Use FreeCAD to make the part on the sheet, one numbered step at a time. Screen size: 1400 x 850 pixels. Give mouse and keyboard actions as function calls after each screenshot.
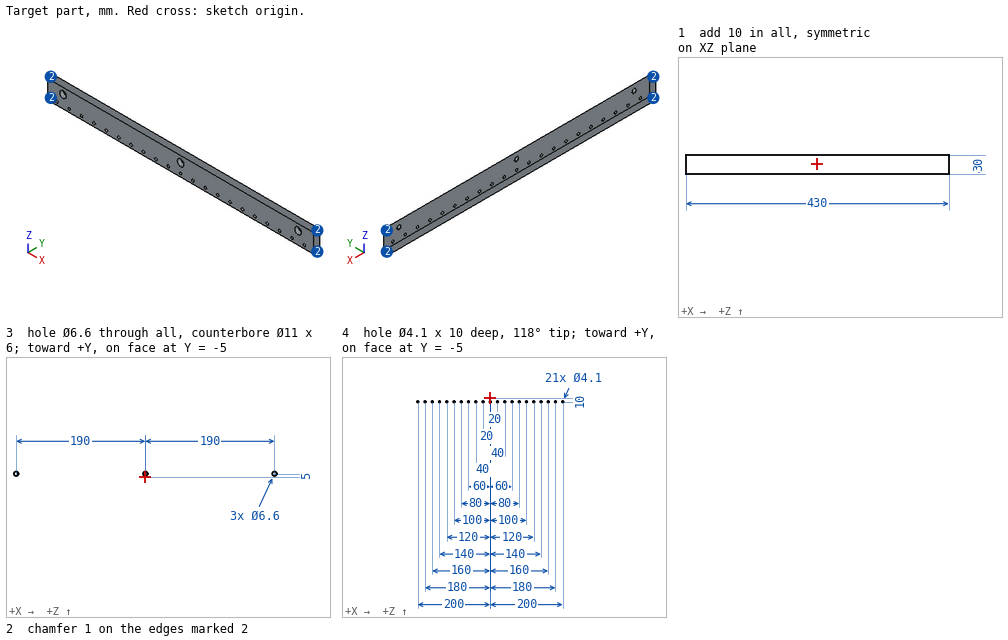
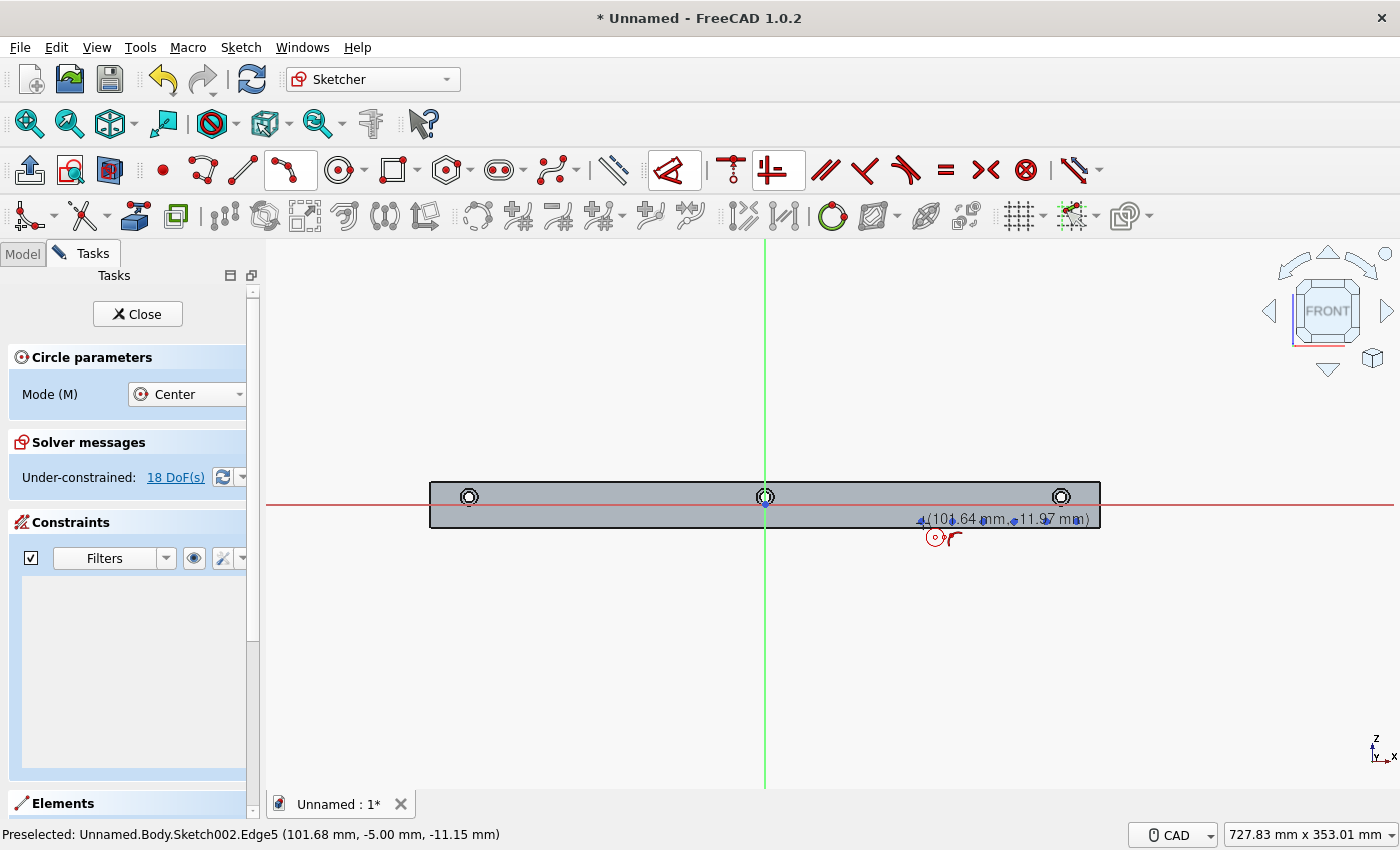
click(890, 521)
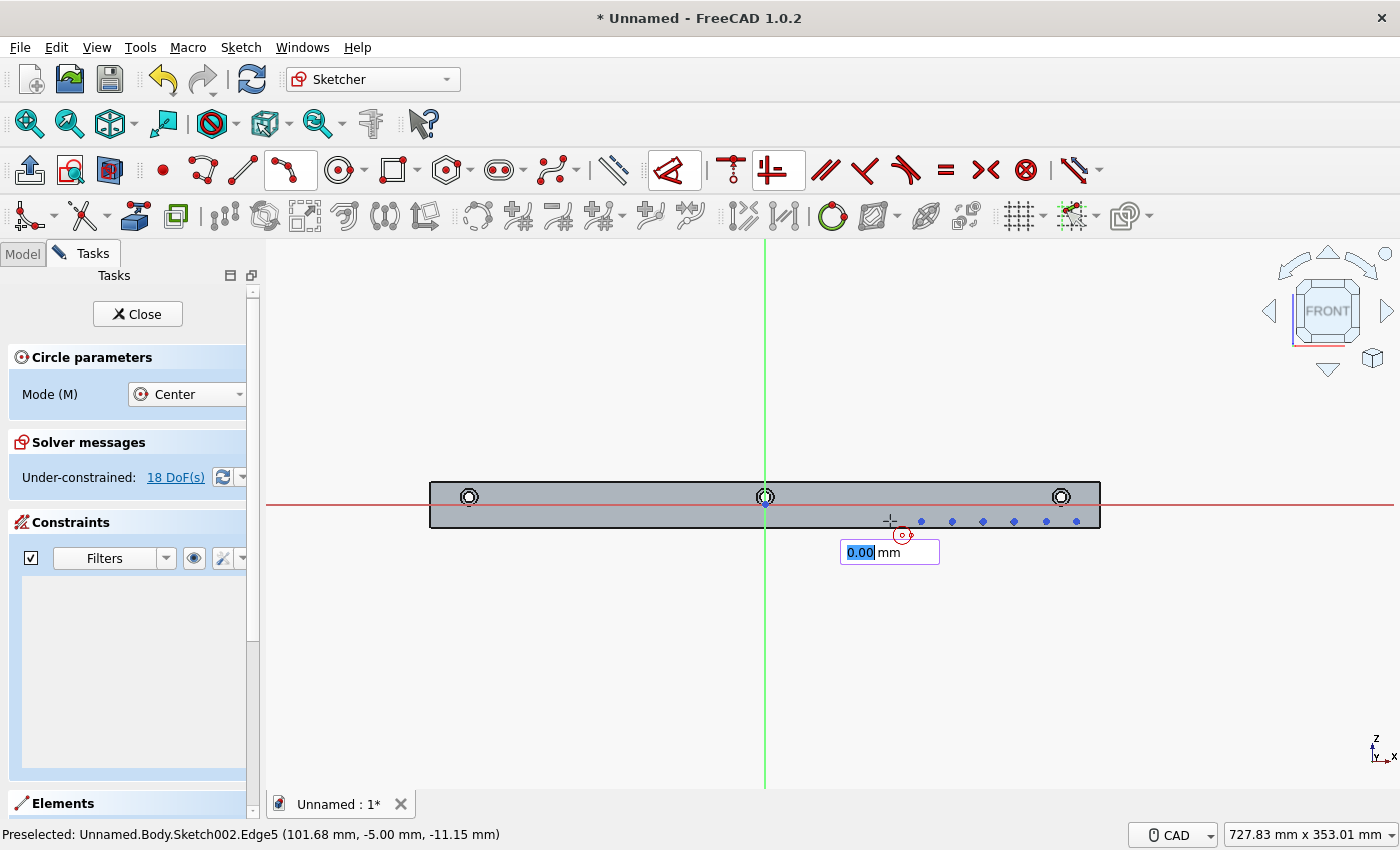
scroll(892, 523, up, 9)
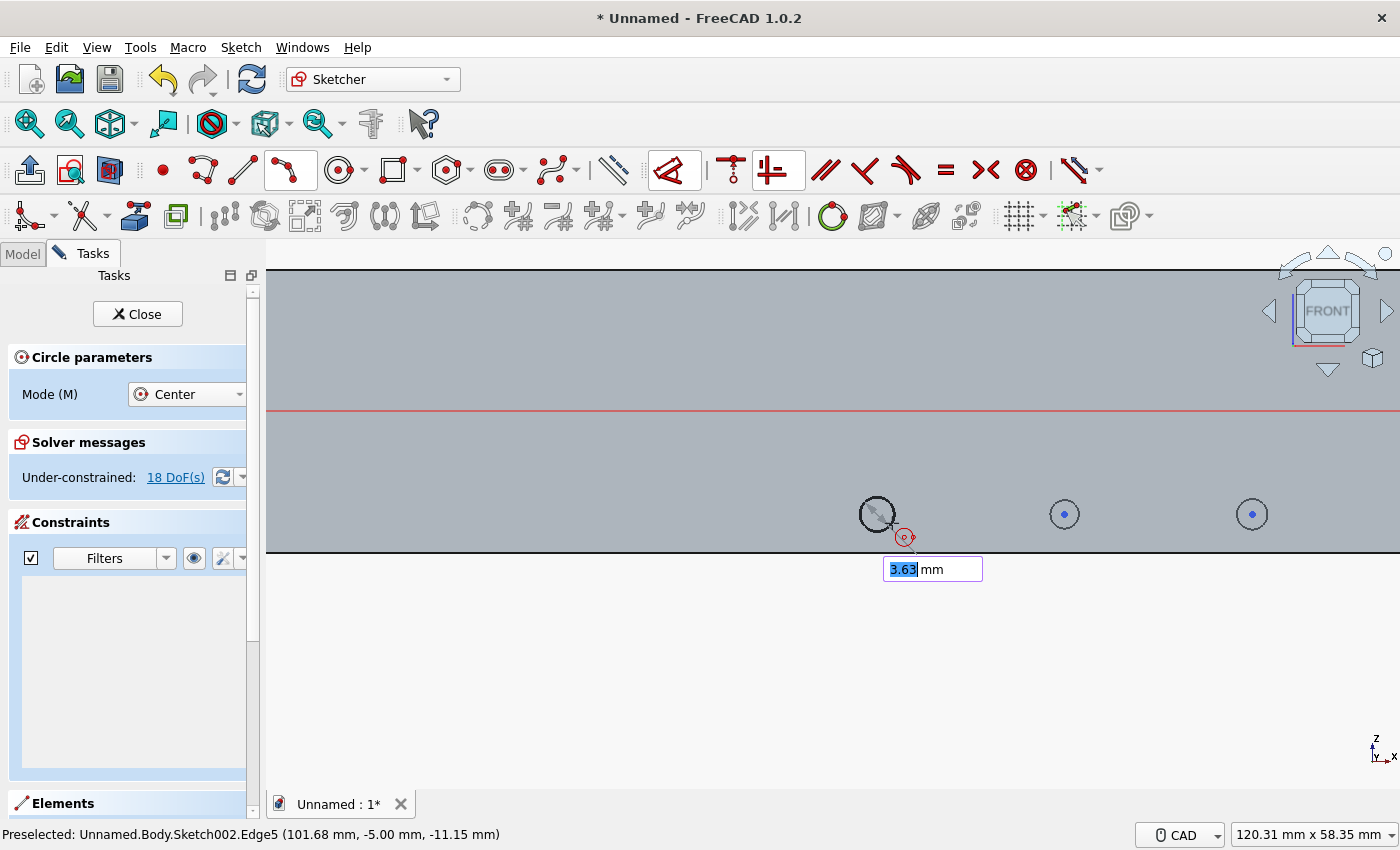
click(889, 519)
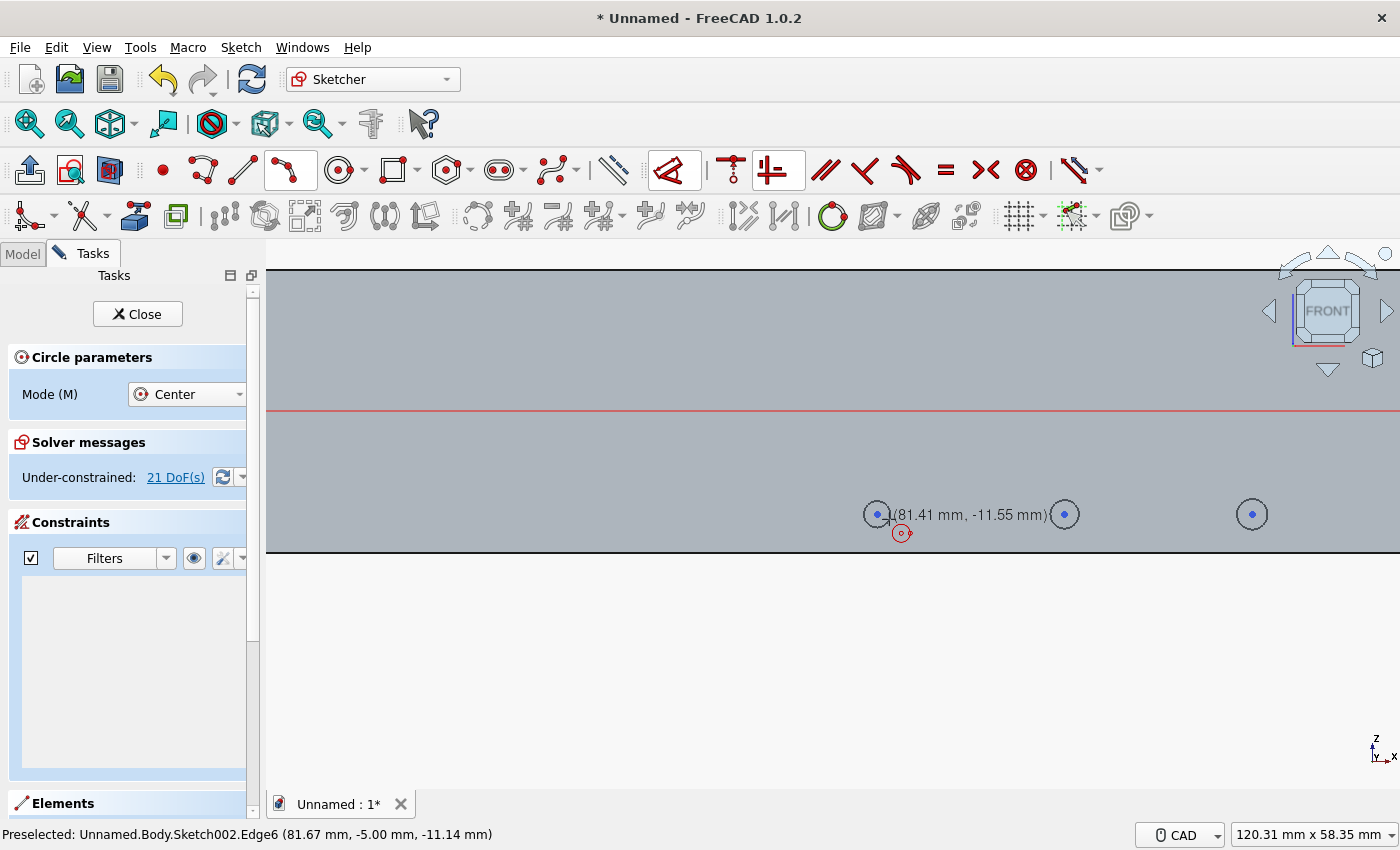
scroll(892, 523, down, 9)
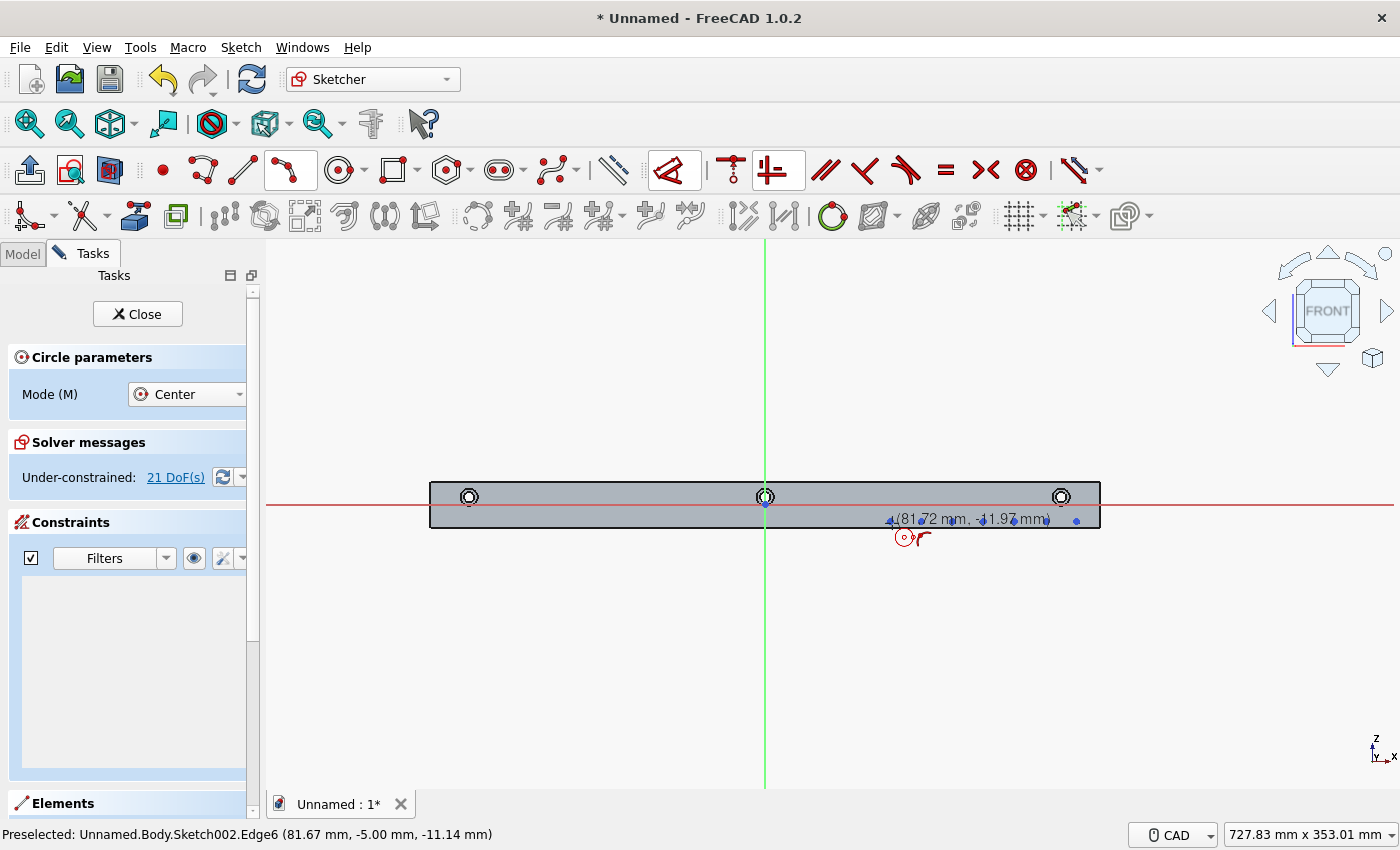
click(859, 521)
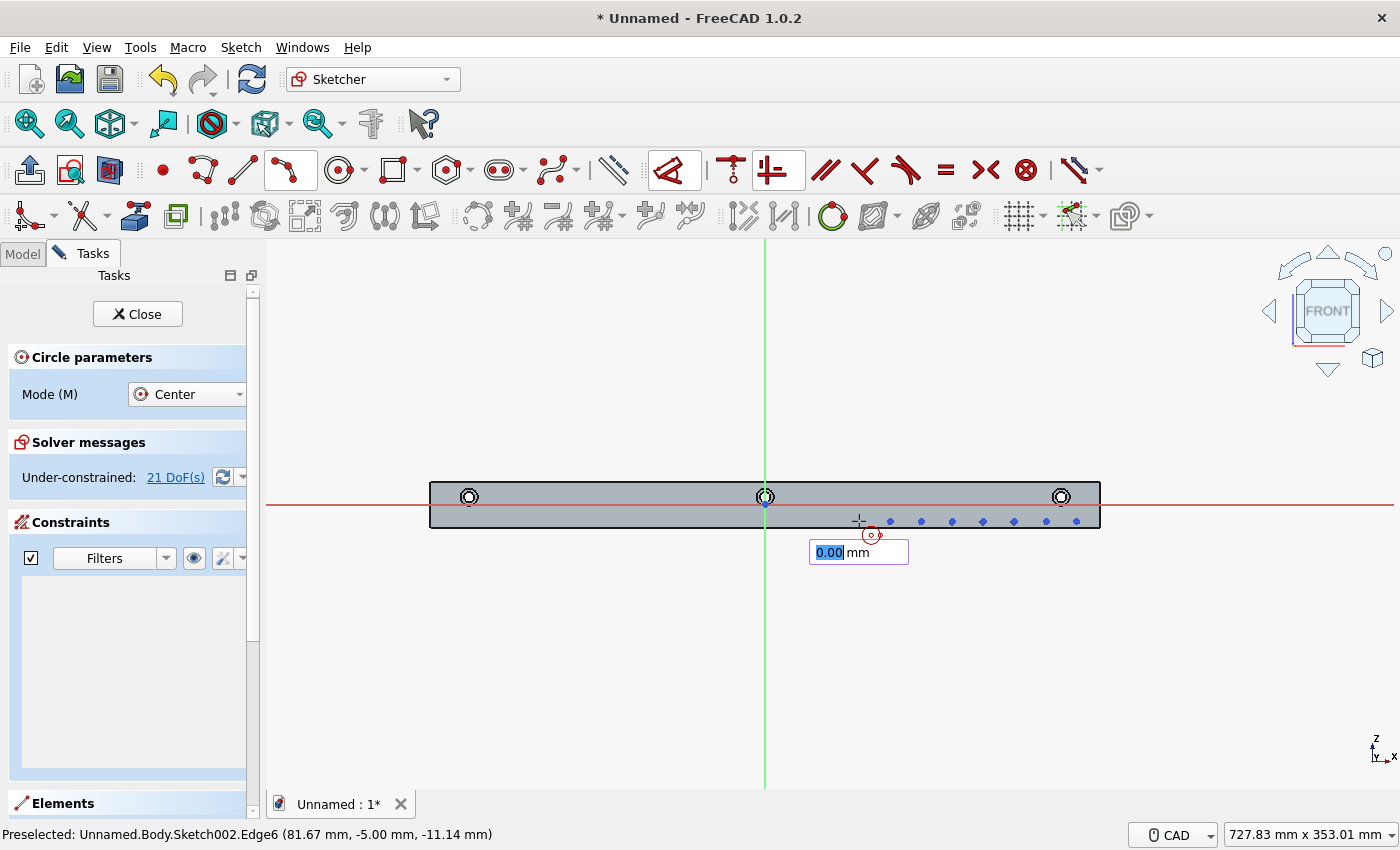
scroll(861, 523, up, 9)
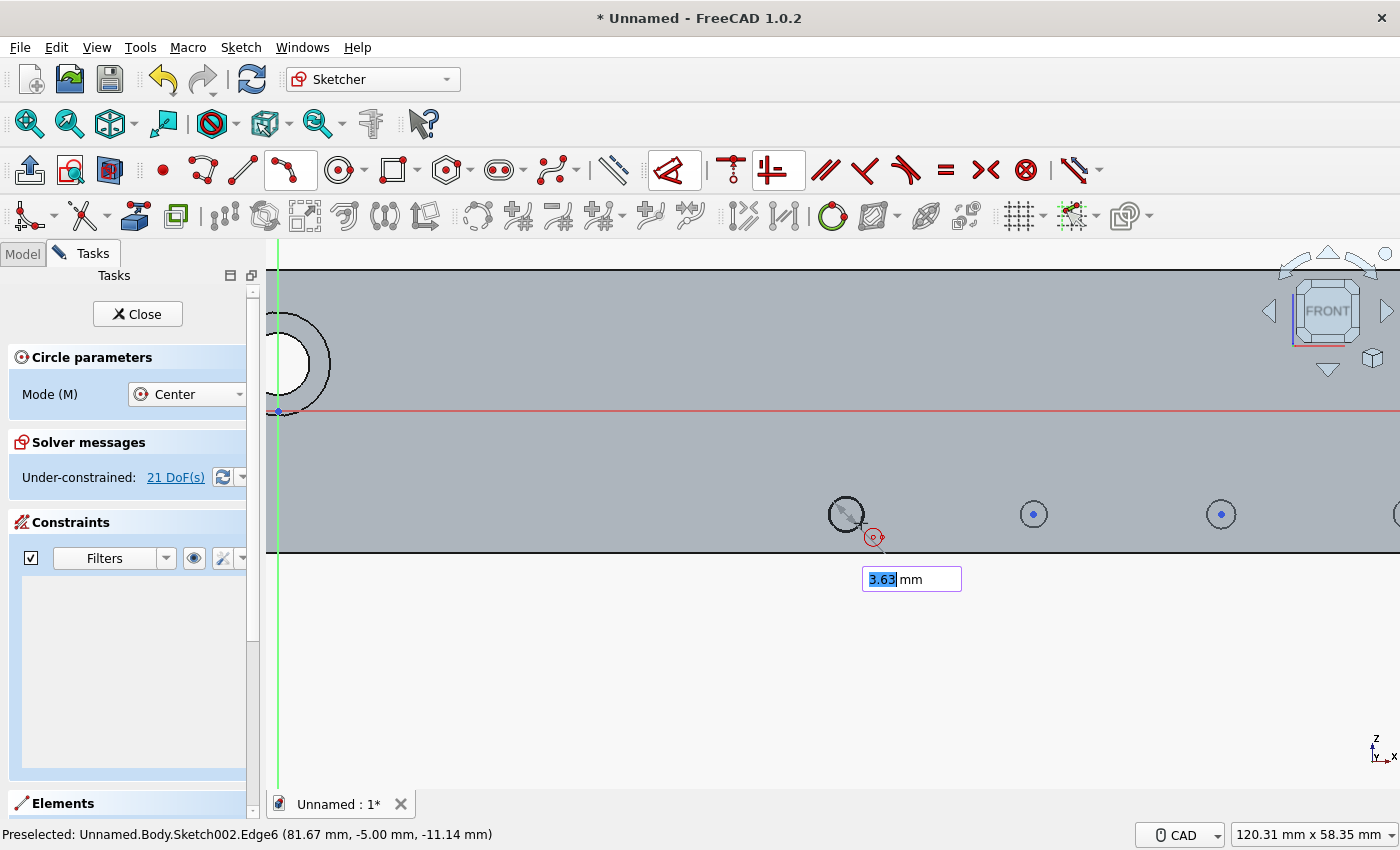
click(858, 519)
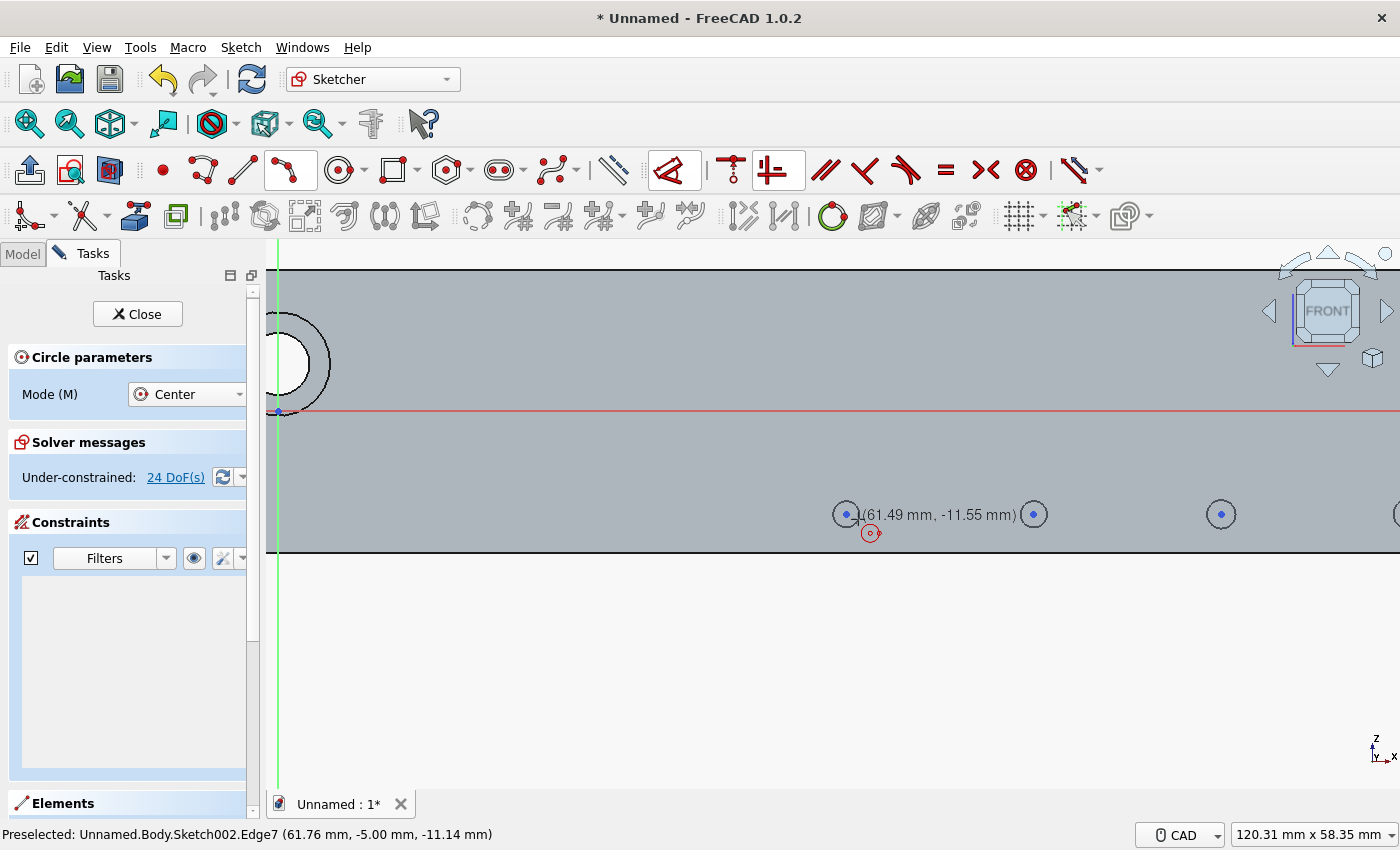
scroll(861, 523, down, 9)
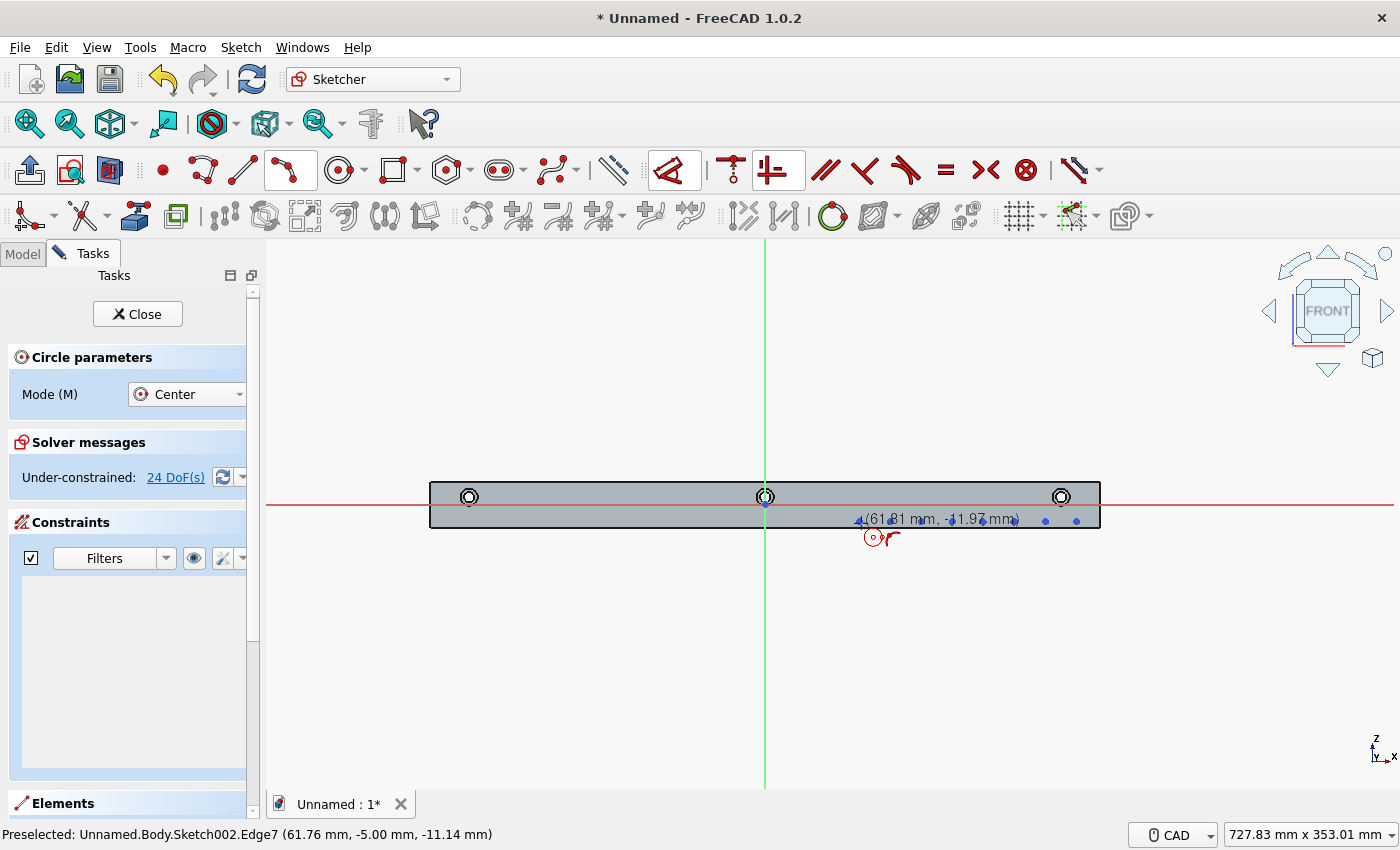
click(827, 521)